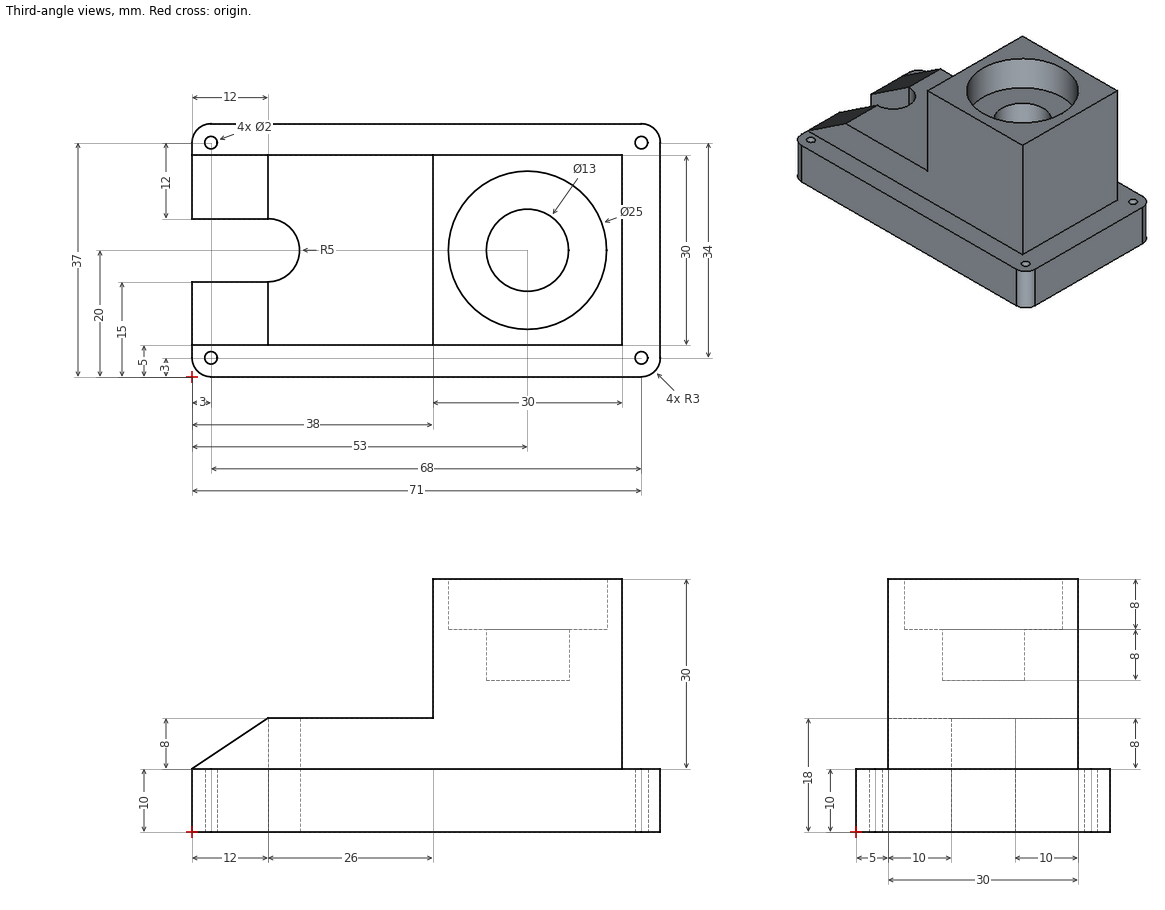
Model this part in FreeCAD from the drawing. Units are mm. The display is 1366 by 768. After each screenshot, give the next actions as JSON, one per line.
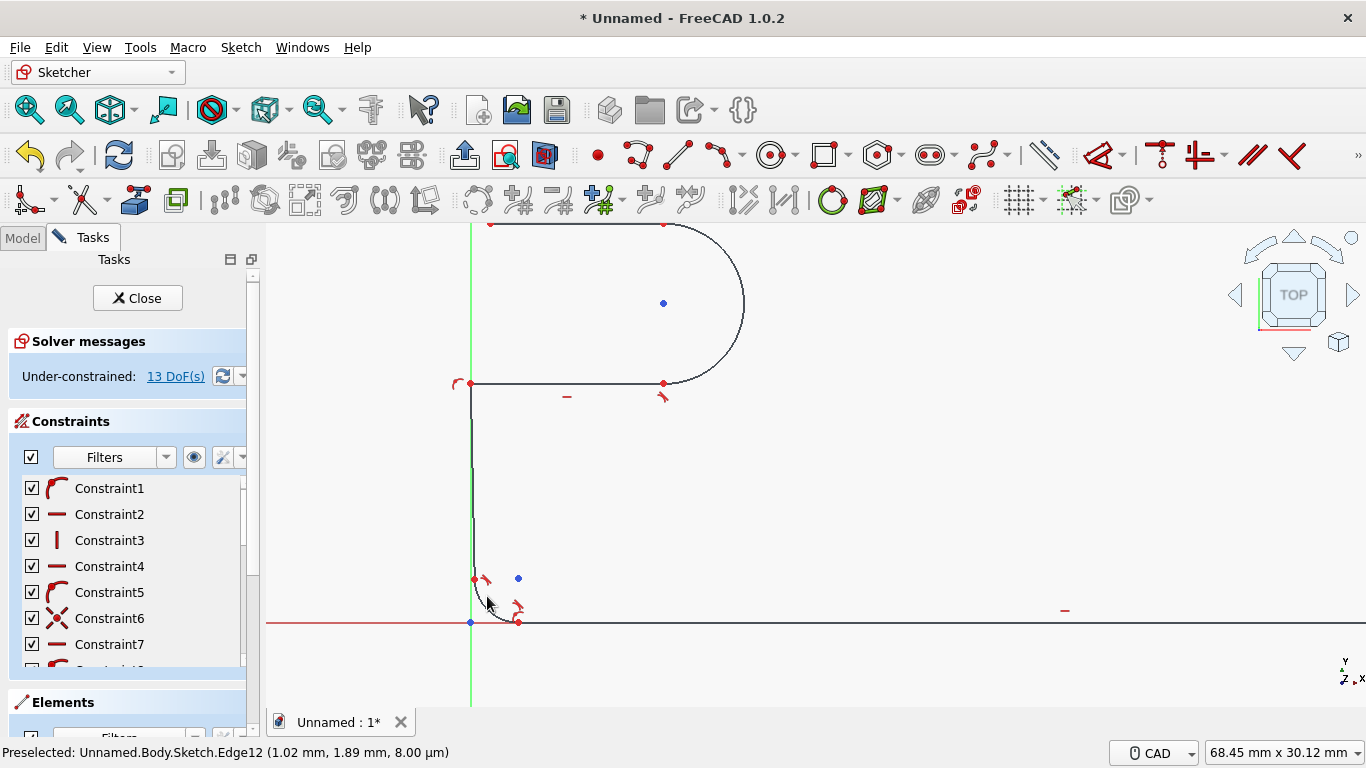
{"action": "scroll", "coordinate": [488, 599], "scroll_direction": "down", "scroll_amount": 4}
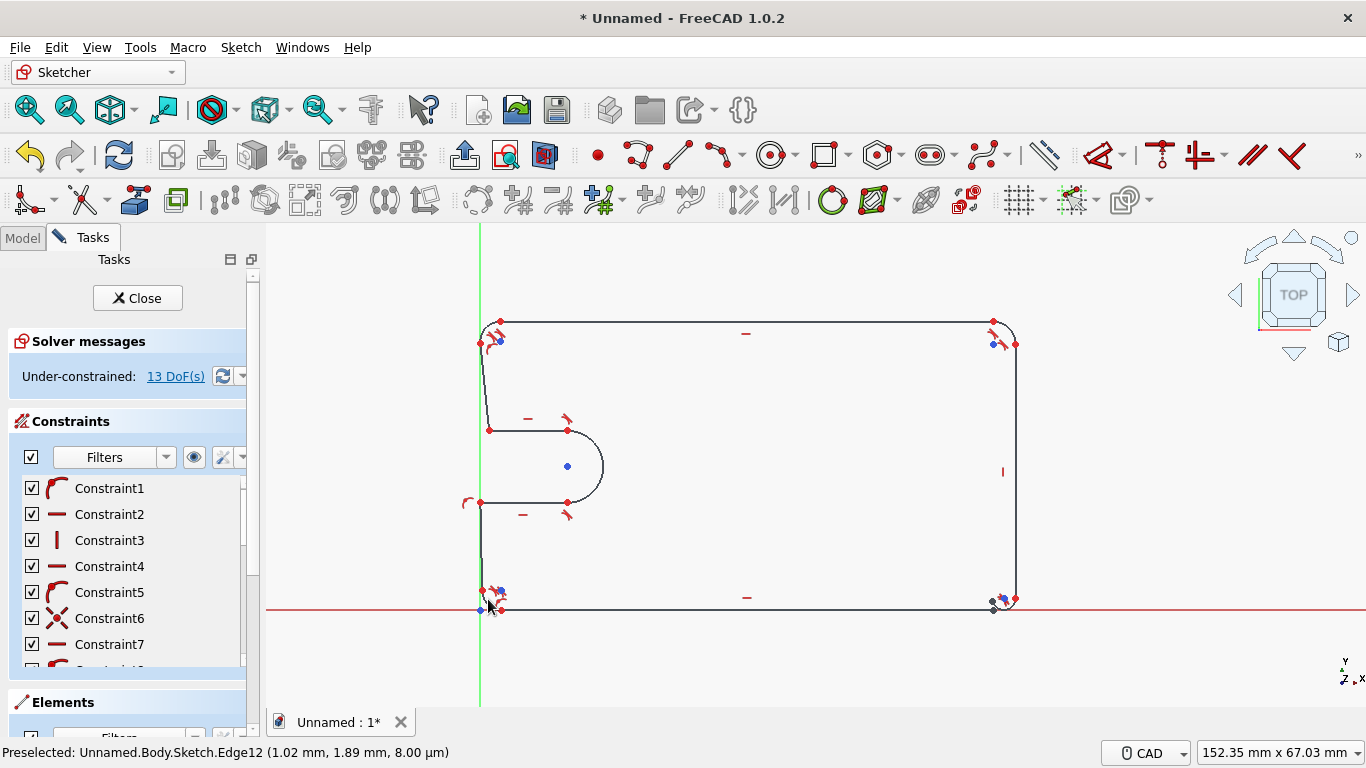
{"action": "scroll", "coordinate": [487, 405], "scroll_direction": "up", "scroll_amount": 5}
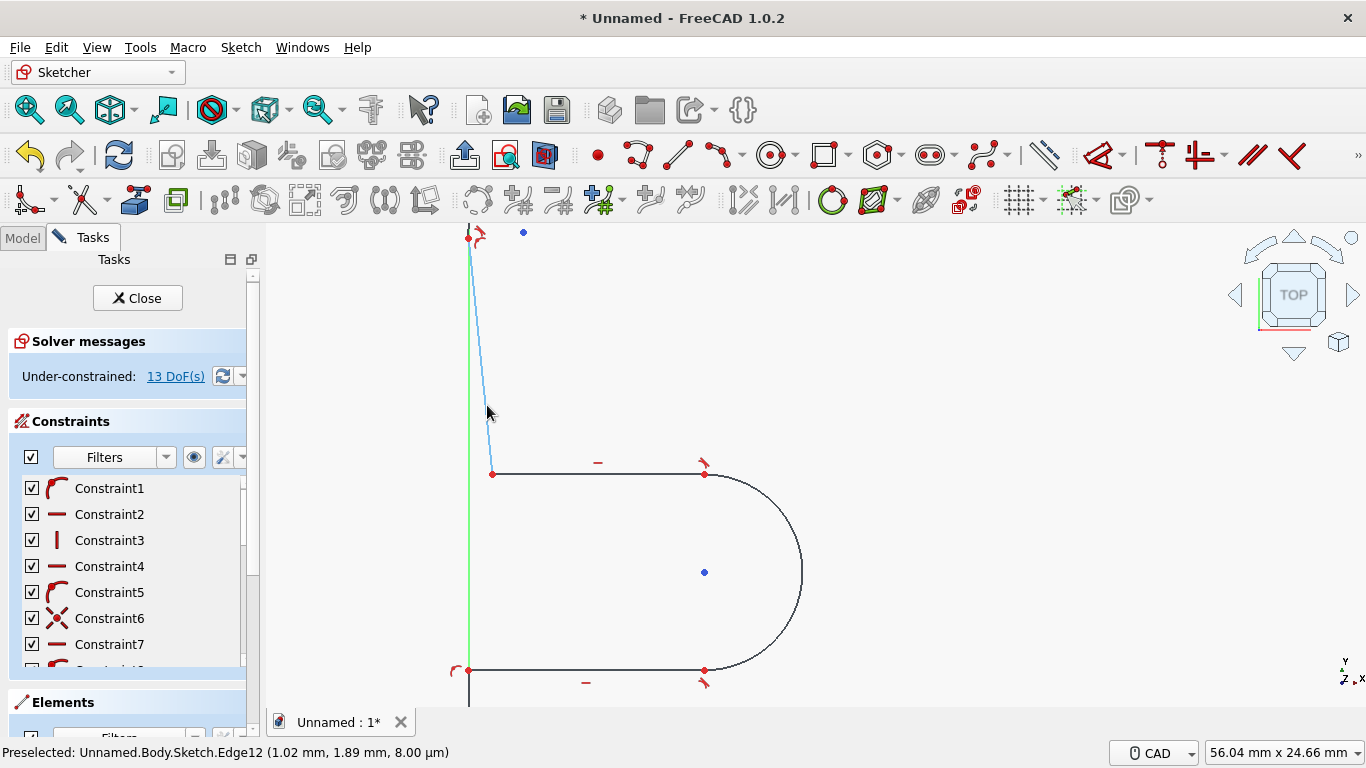
{"action": "left_click", "coordinate": [485, 404]}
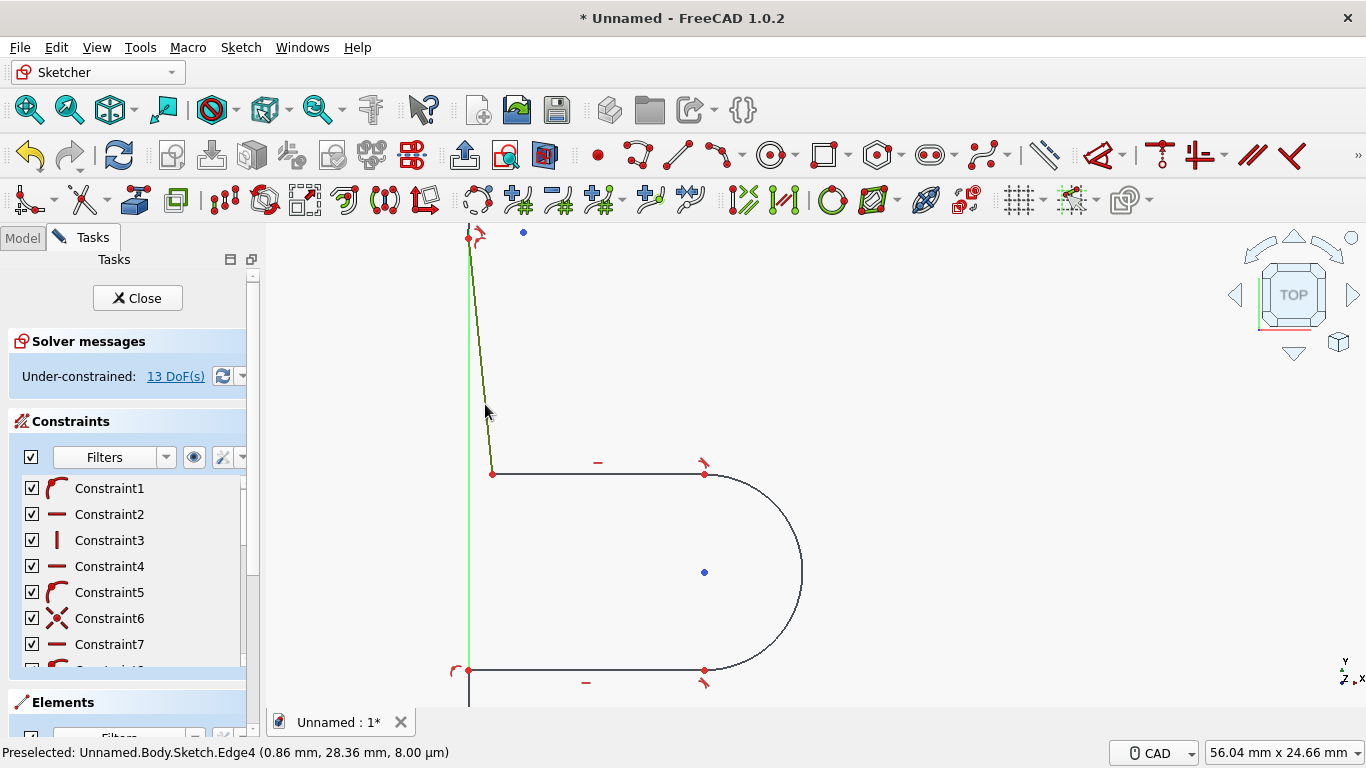
{"action": "key", "text": "v"}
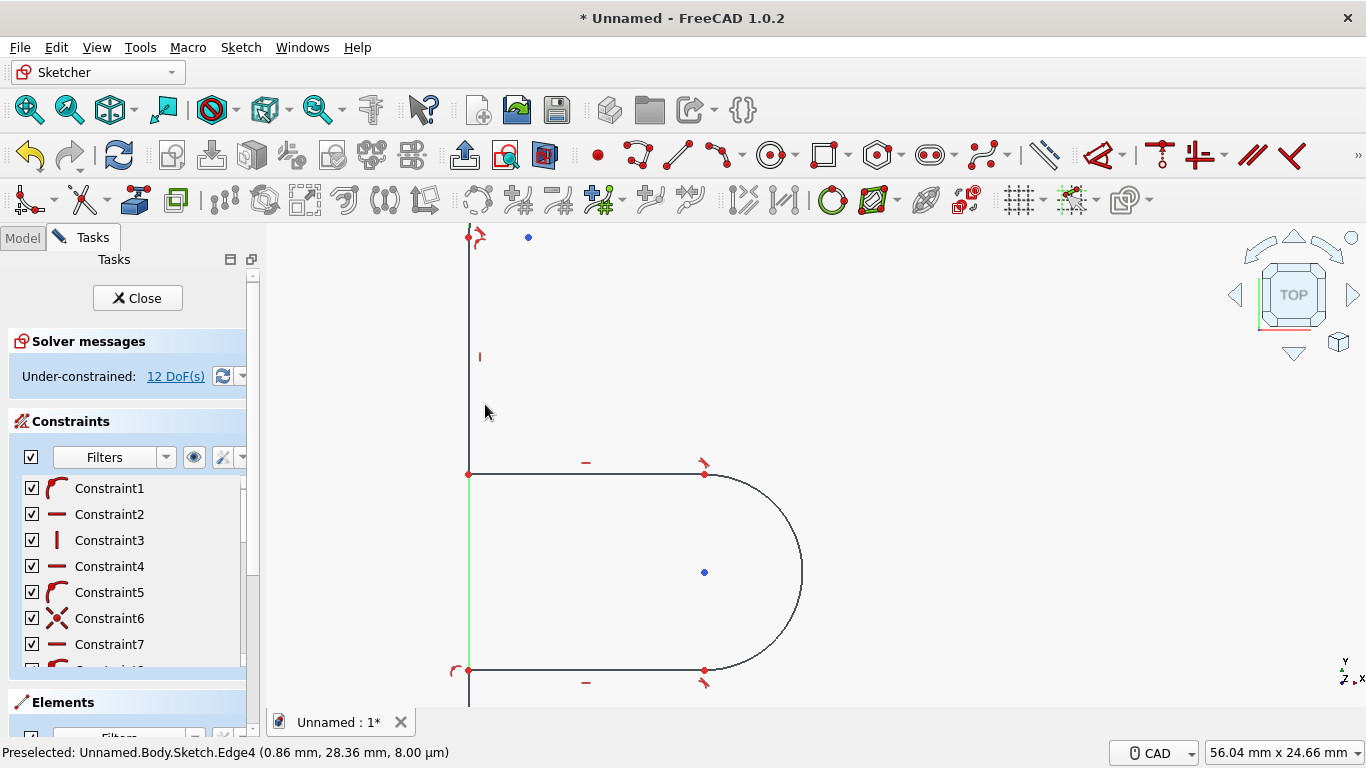
{"action": "scroll", "coordinate": [487, 404], "scroll_direction": "down", "scroll_amount": 5}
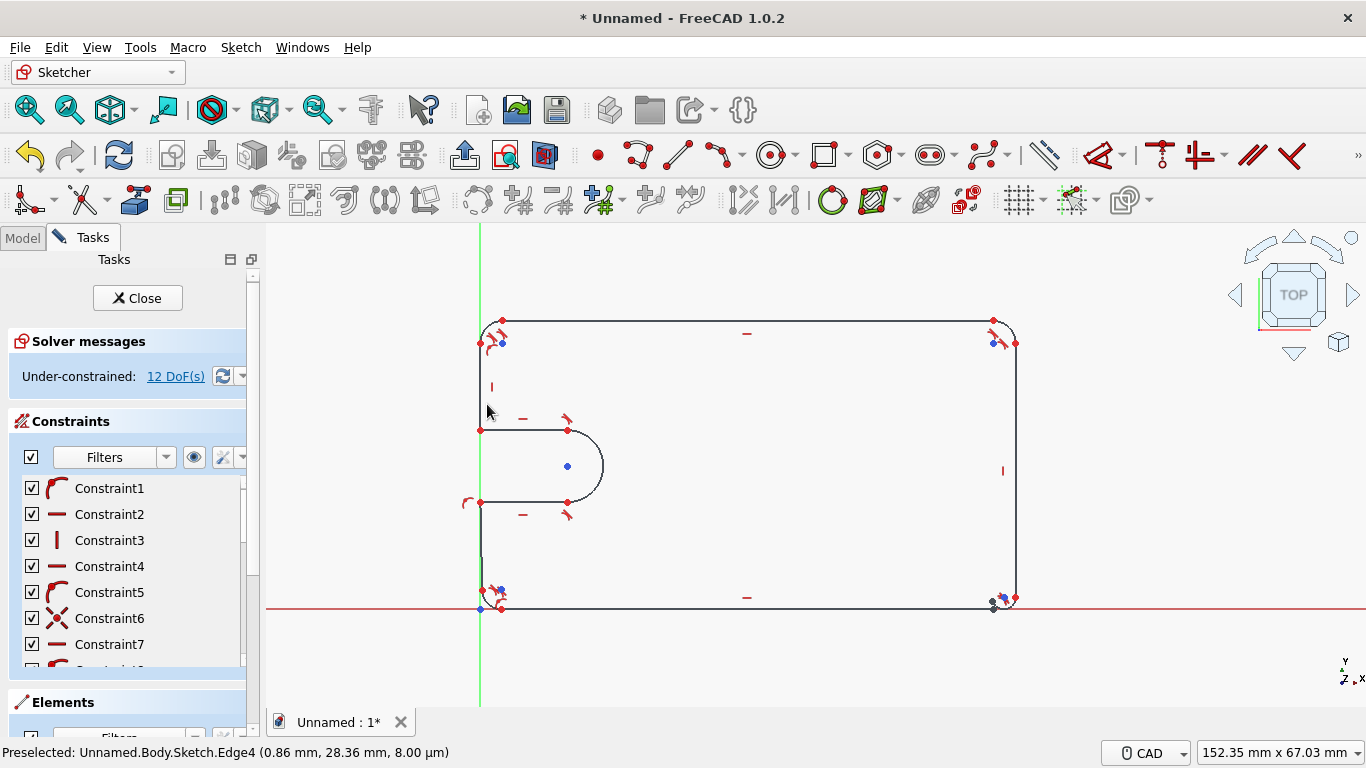
{"action": "left_click", "coordinate": [481, 529]}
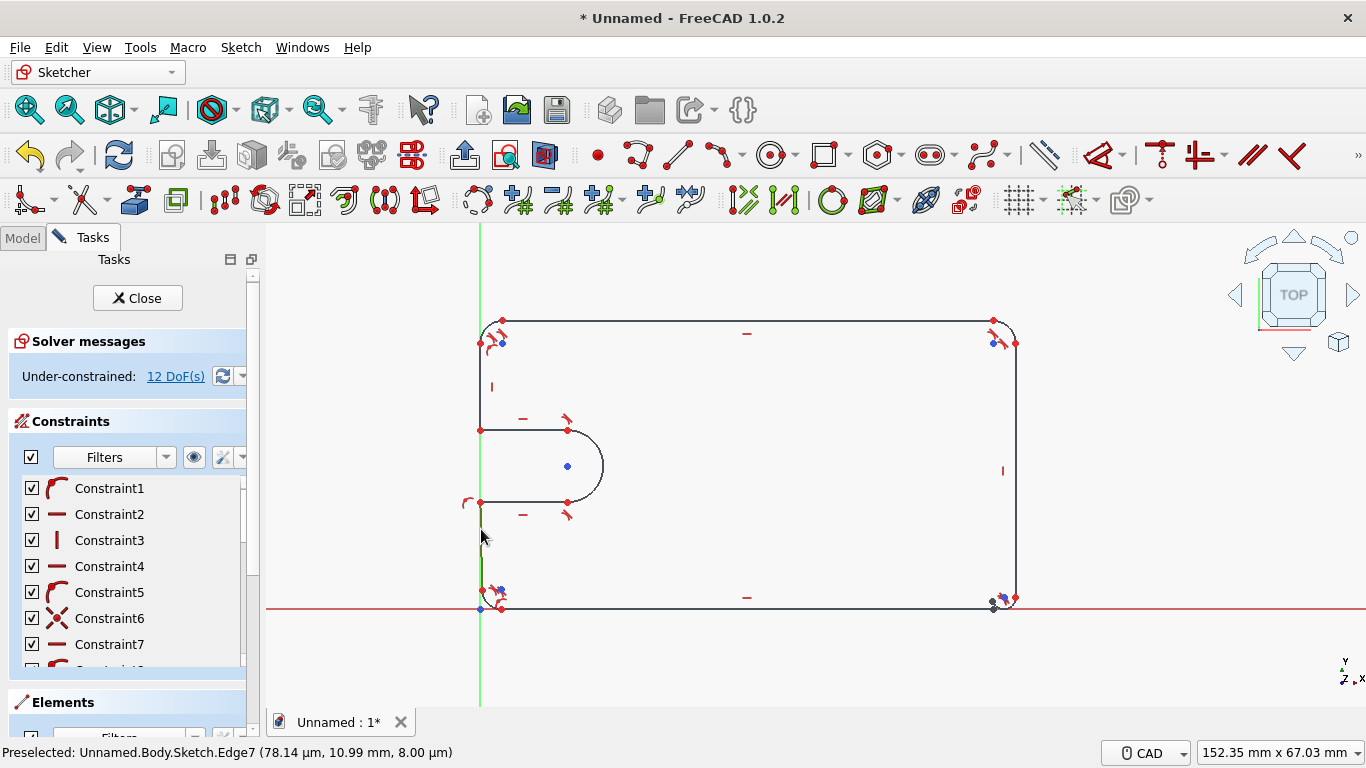
{"action": "key", "text": "v"}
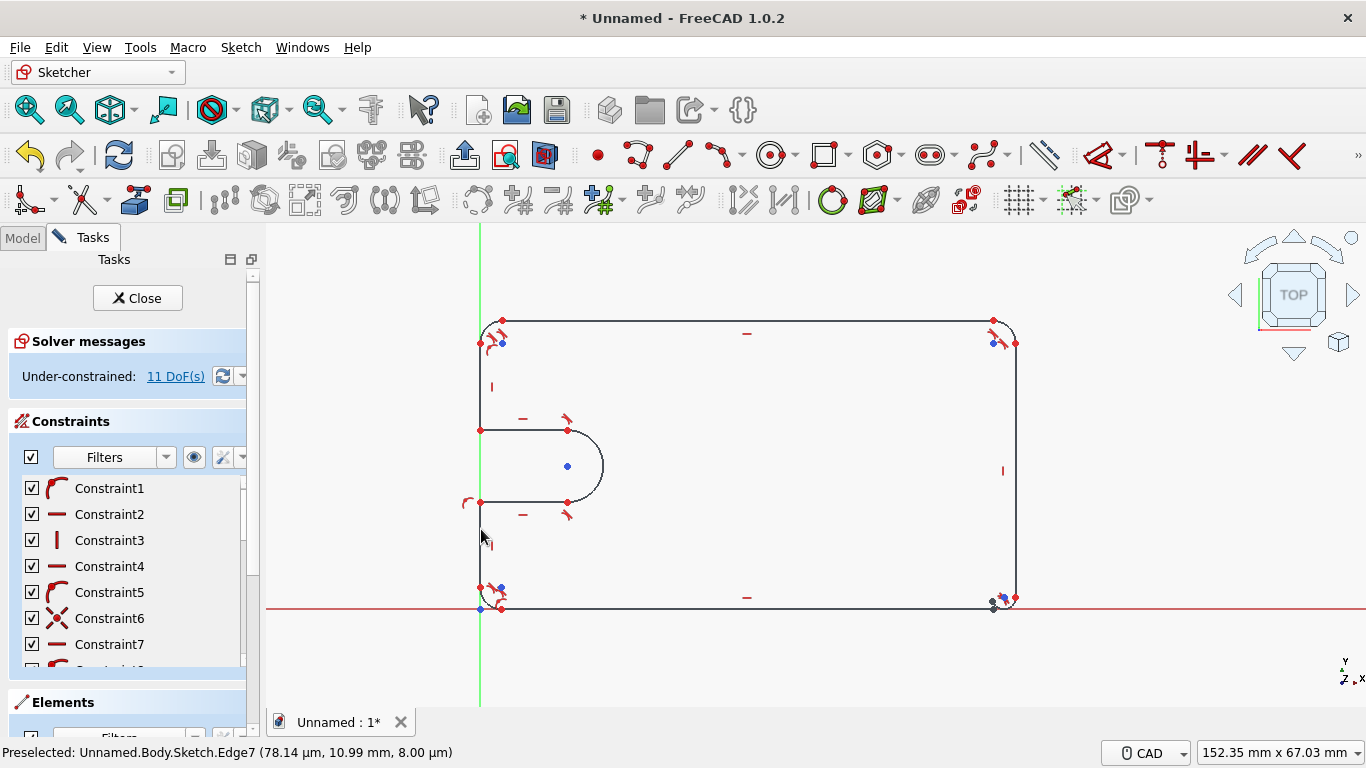
{"action": "scroll", "coordinate": [1012, 607], "scroll_direction": "up", "scroll_amount": 2}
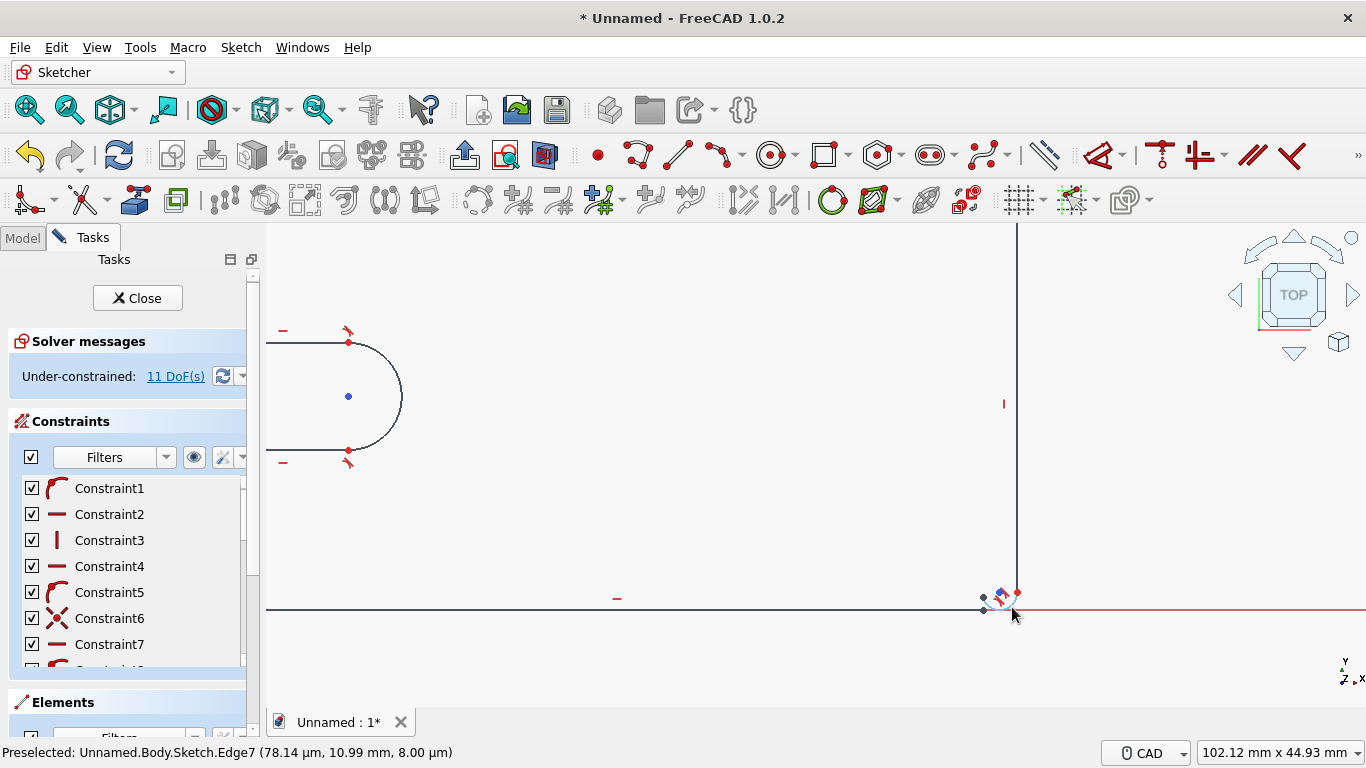
{"action": "left_click", "coordinate": [1011, 606]}